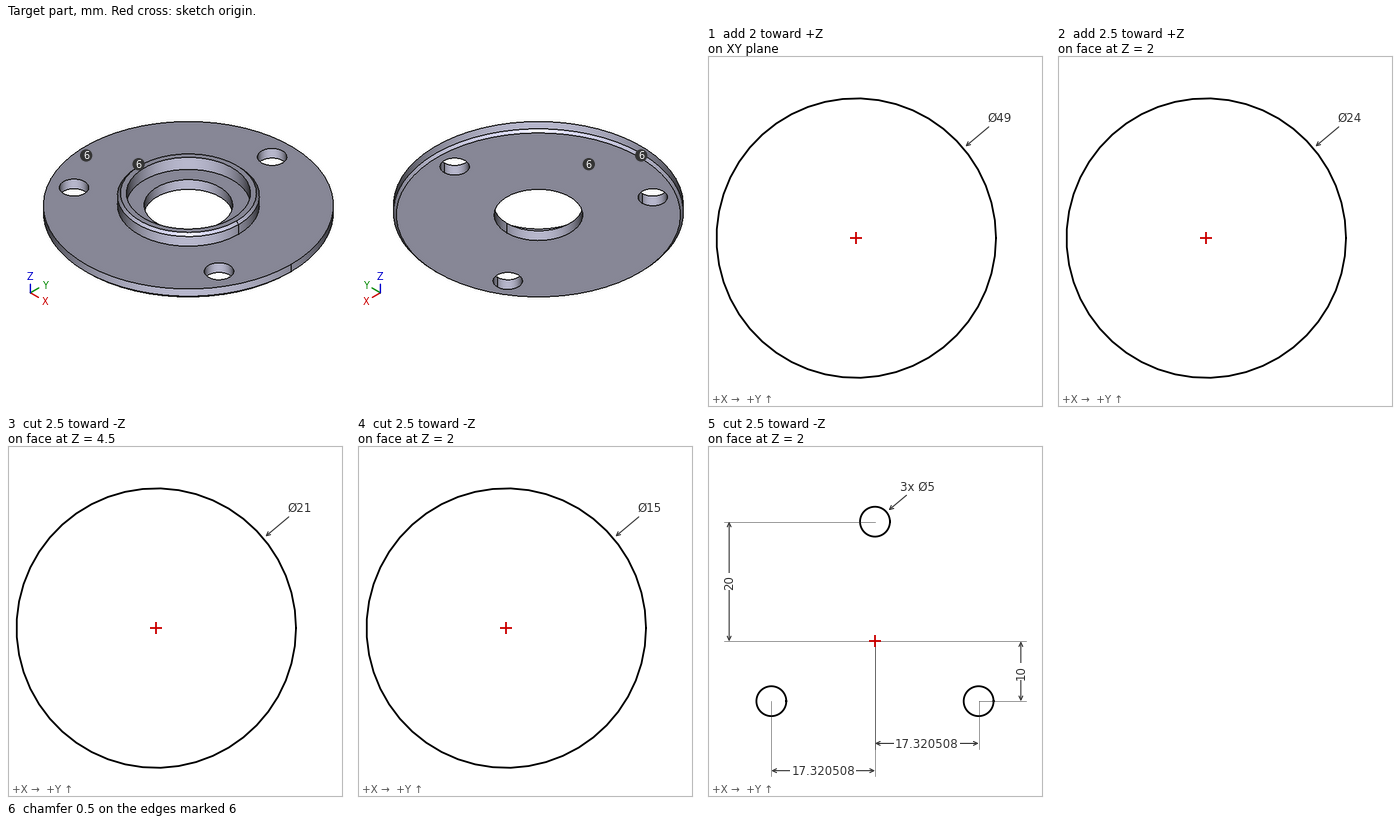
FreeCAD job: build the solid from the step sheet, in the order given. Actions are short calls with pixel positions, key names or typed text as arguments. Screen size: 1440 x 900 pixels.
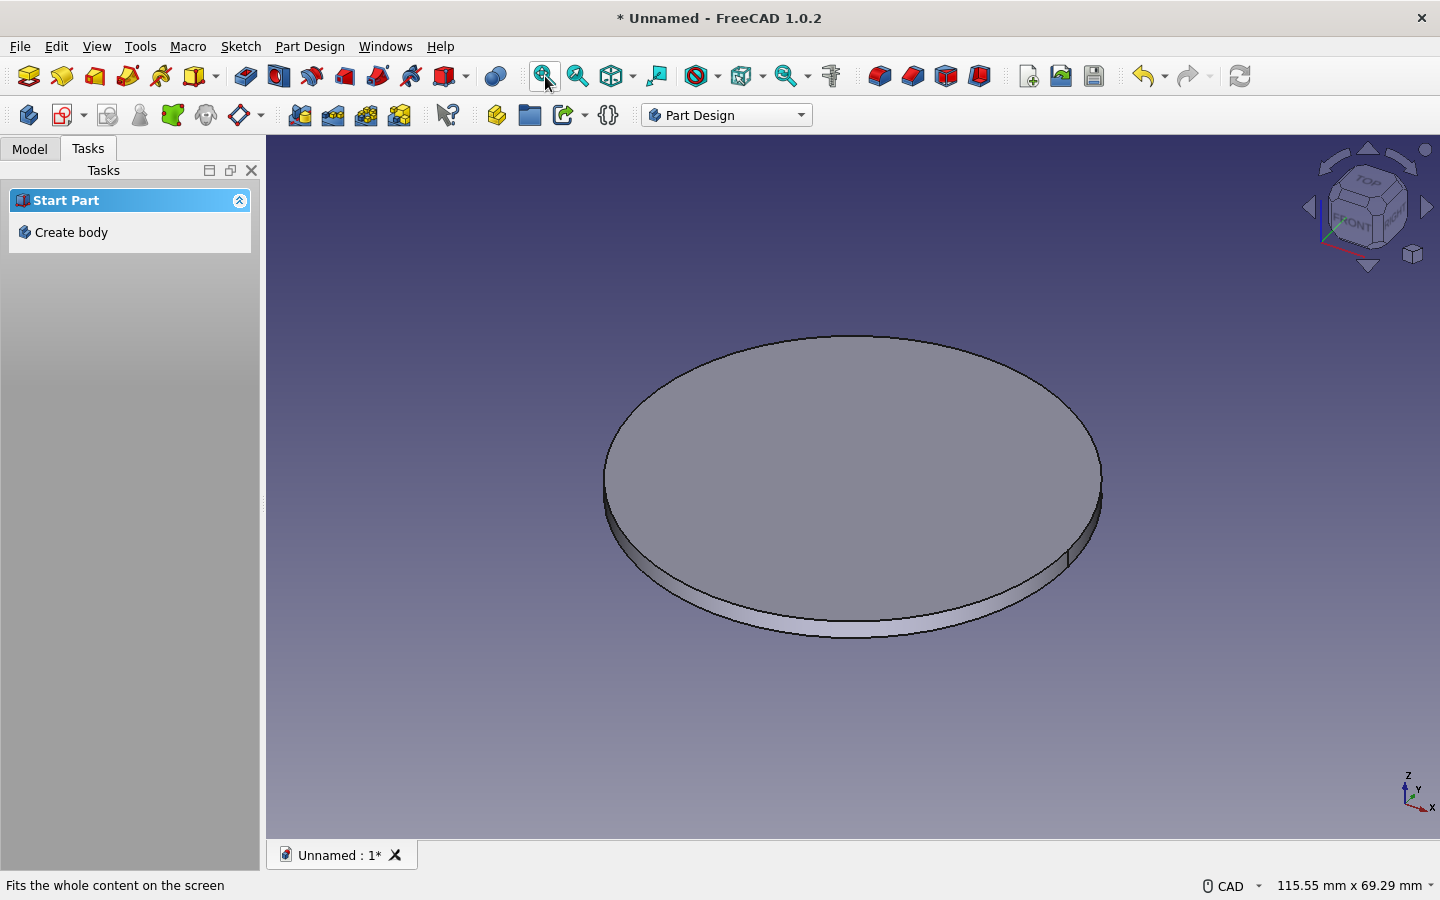
click(853, 478)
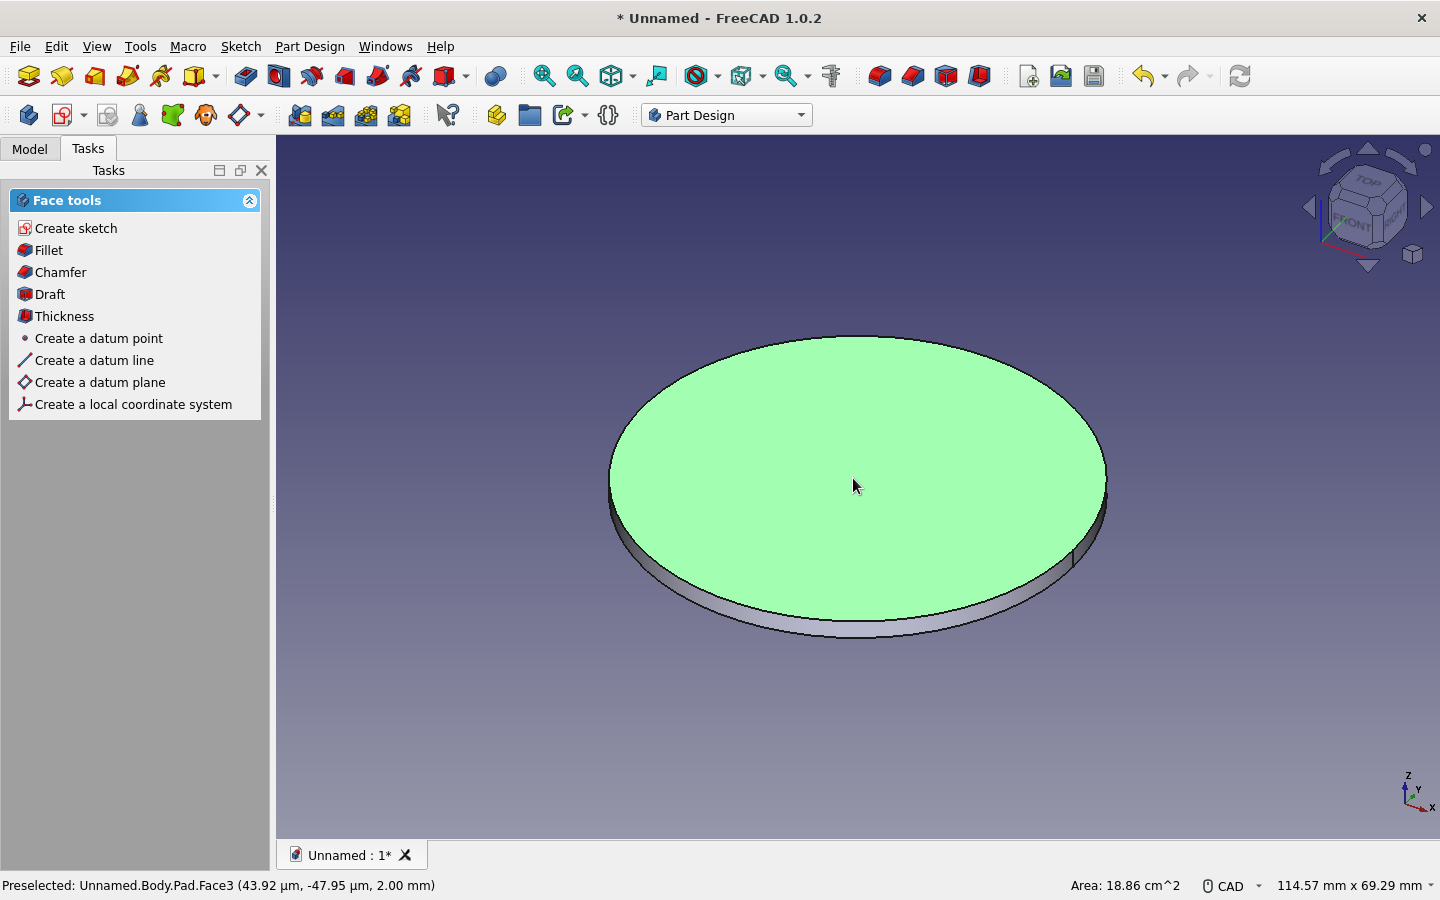
click(62, 116)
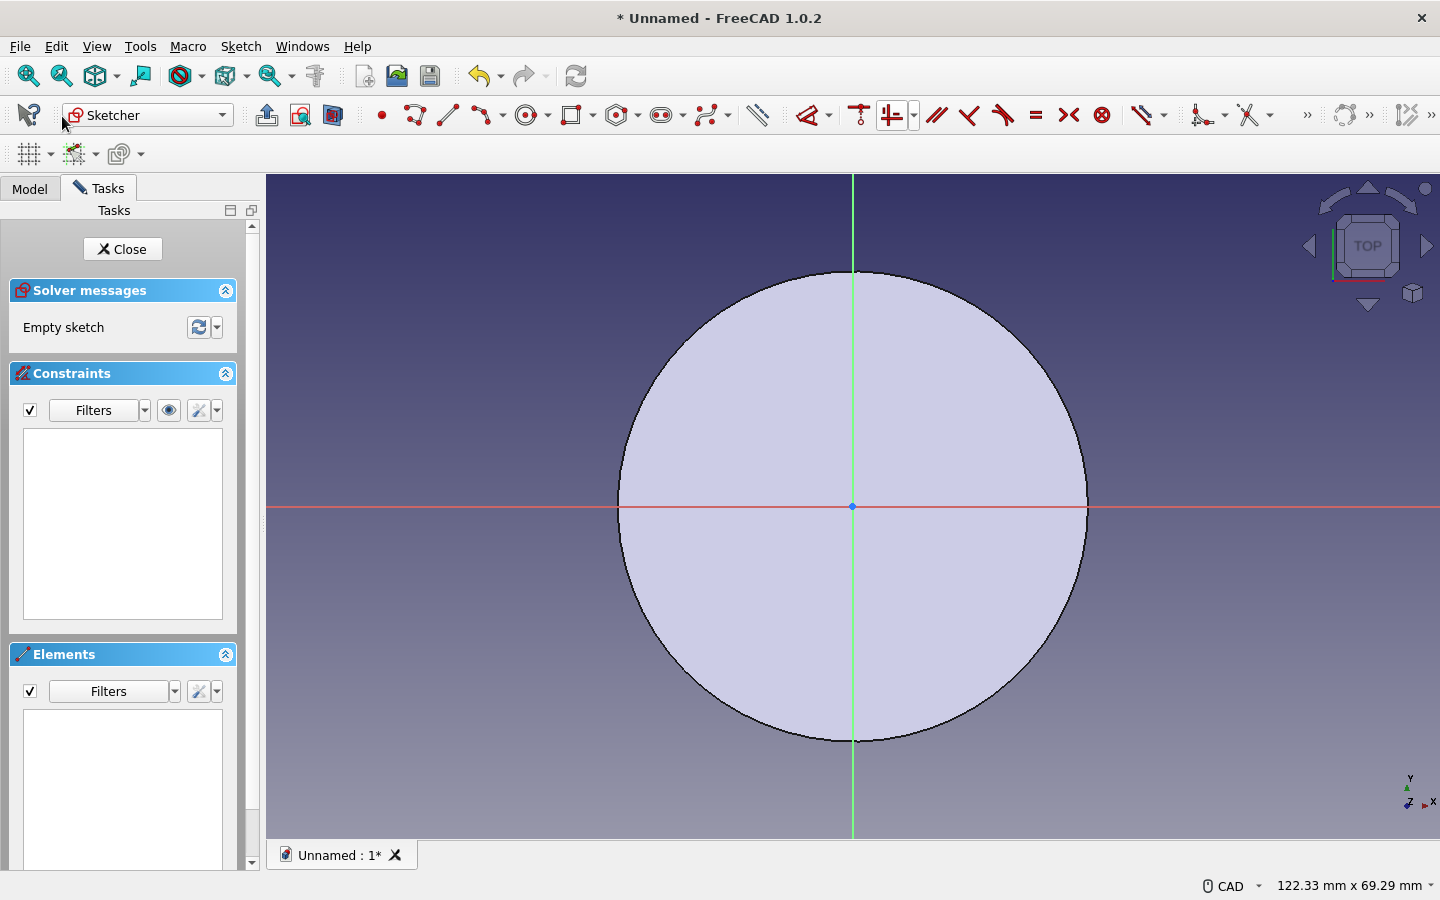
scroll(936, 507, up, 3)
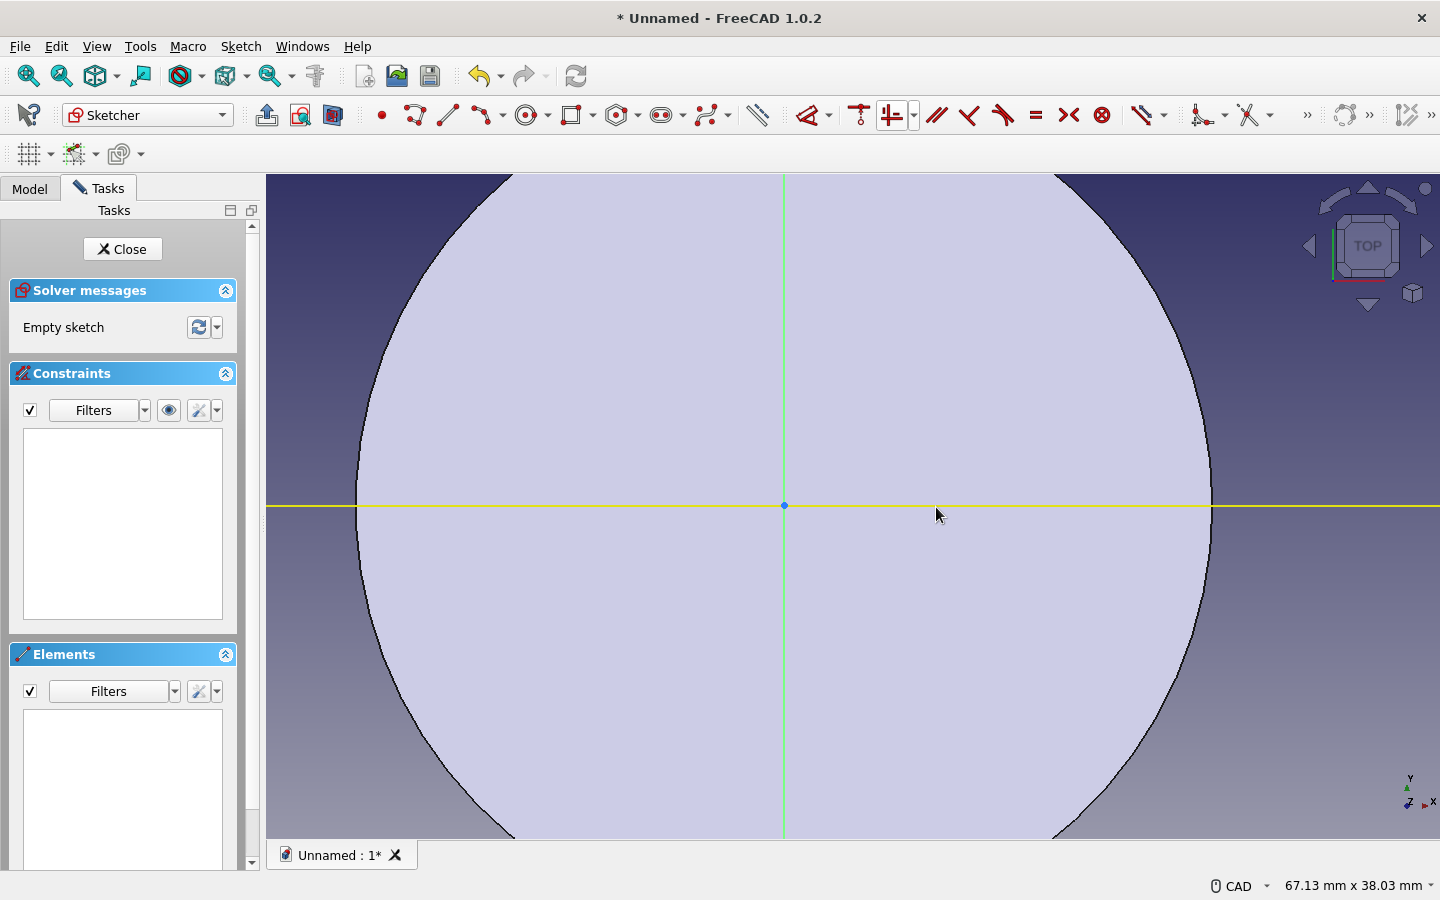
click(526, 116)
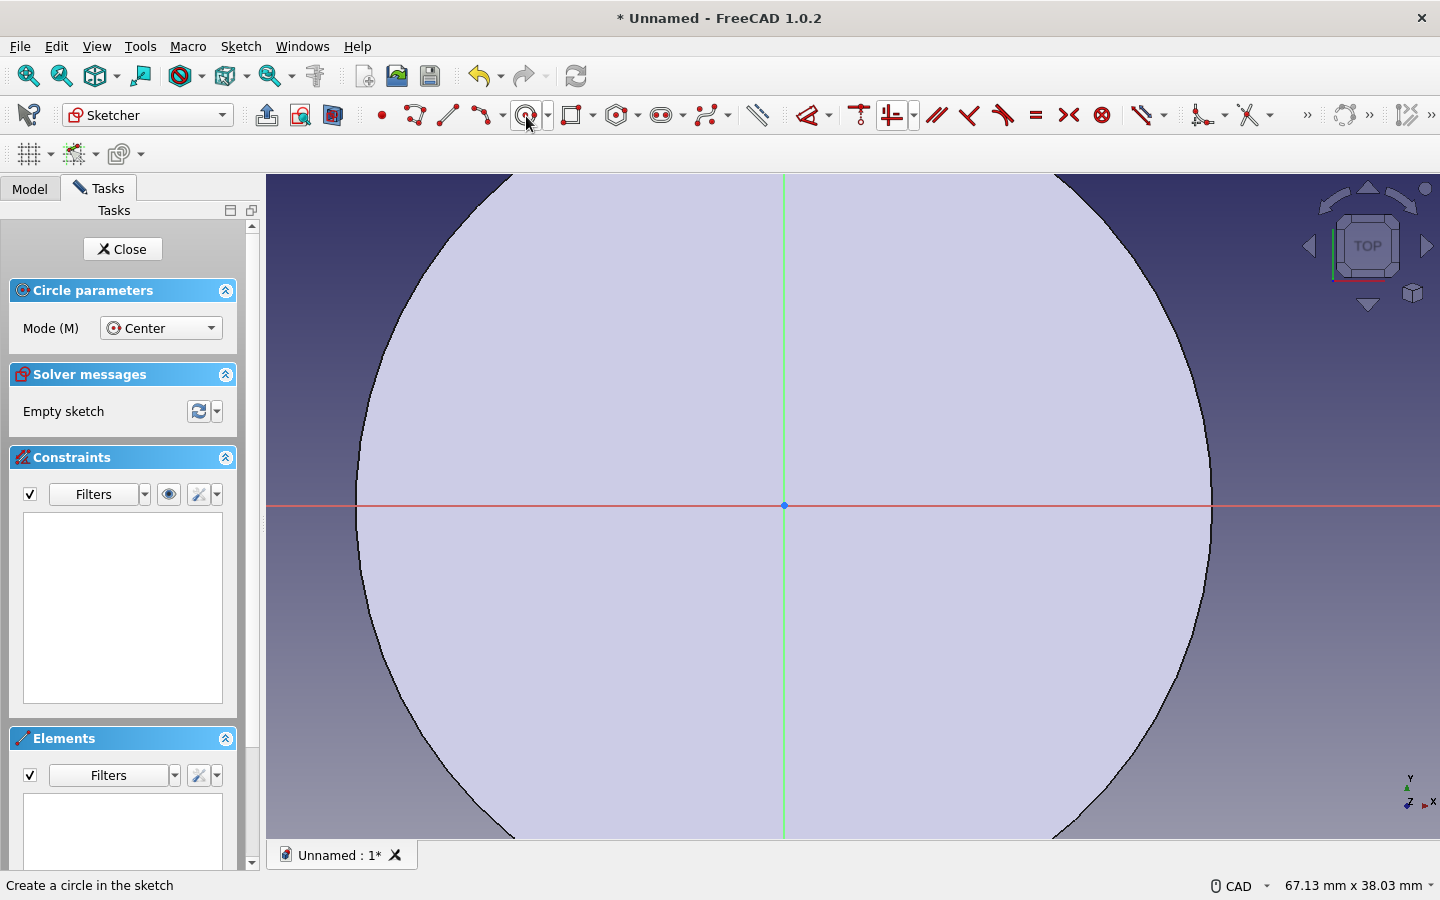
click(784, 506)
click(932, 357)
key(Escape)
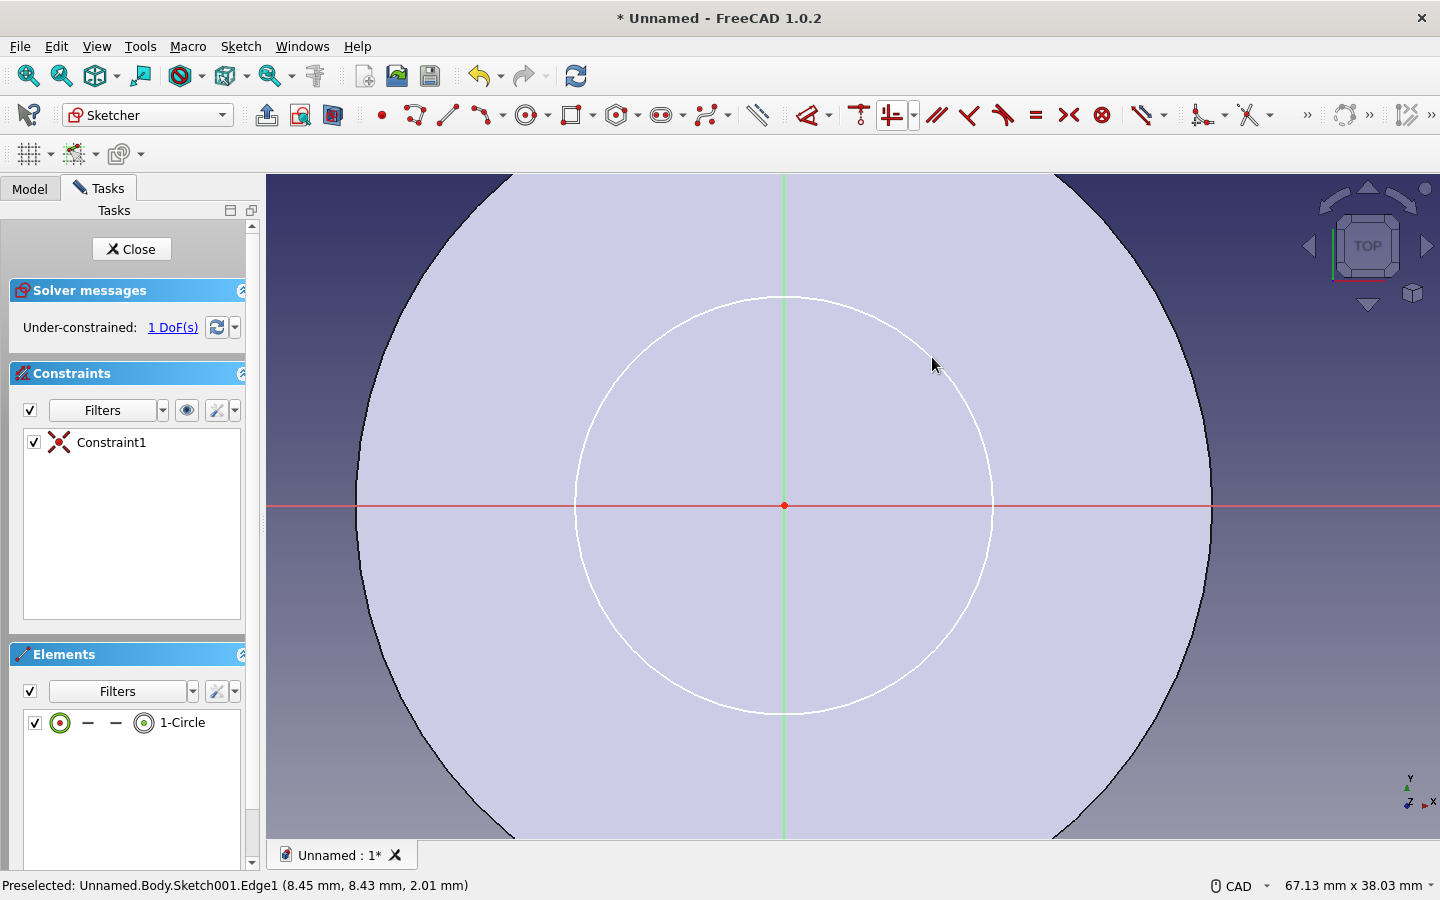
click(931, 357)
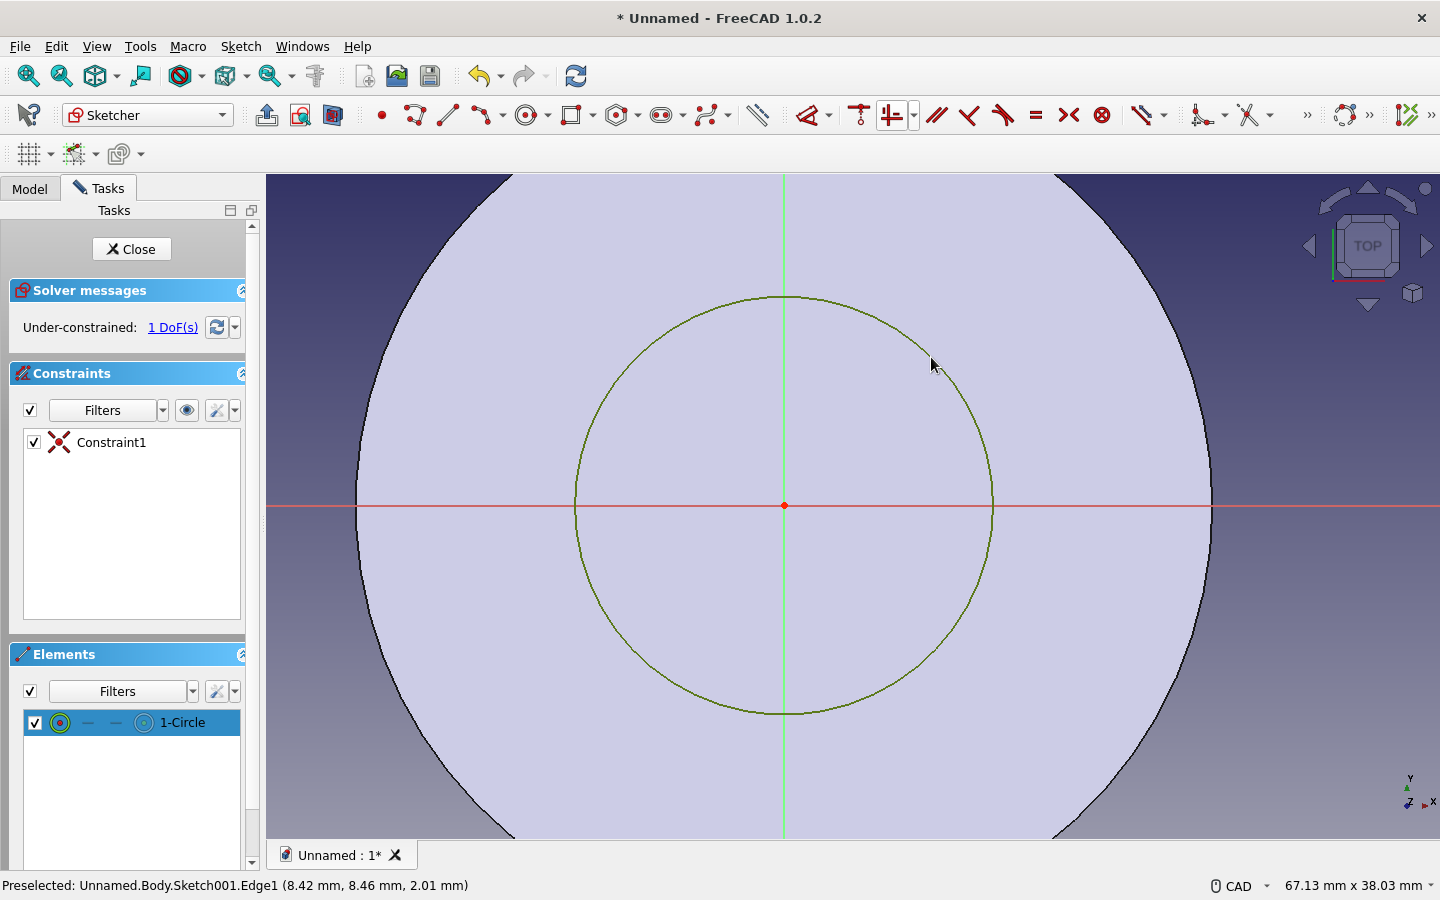
key(k)
key(o)